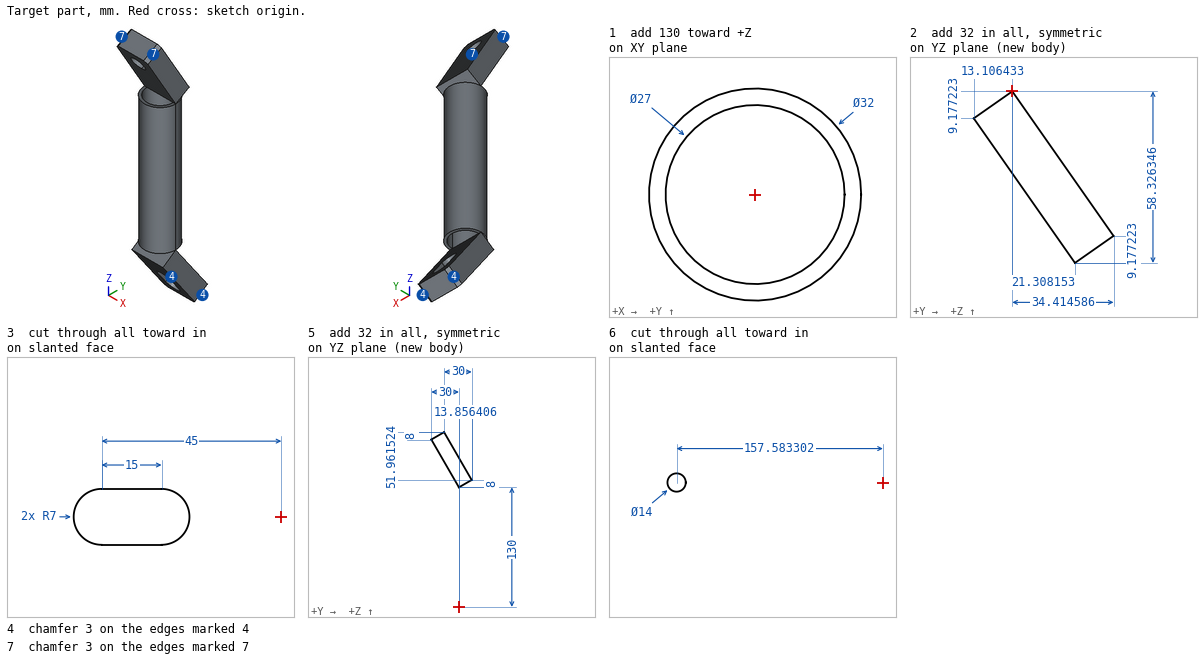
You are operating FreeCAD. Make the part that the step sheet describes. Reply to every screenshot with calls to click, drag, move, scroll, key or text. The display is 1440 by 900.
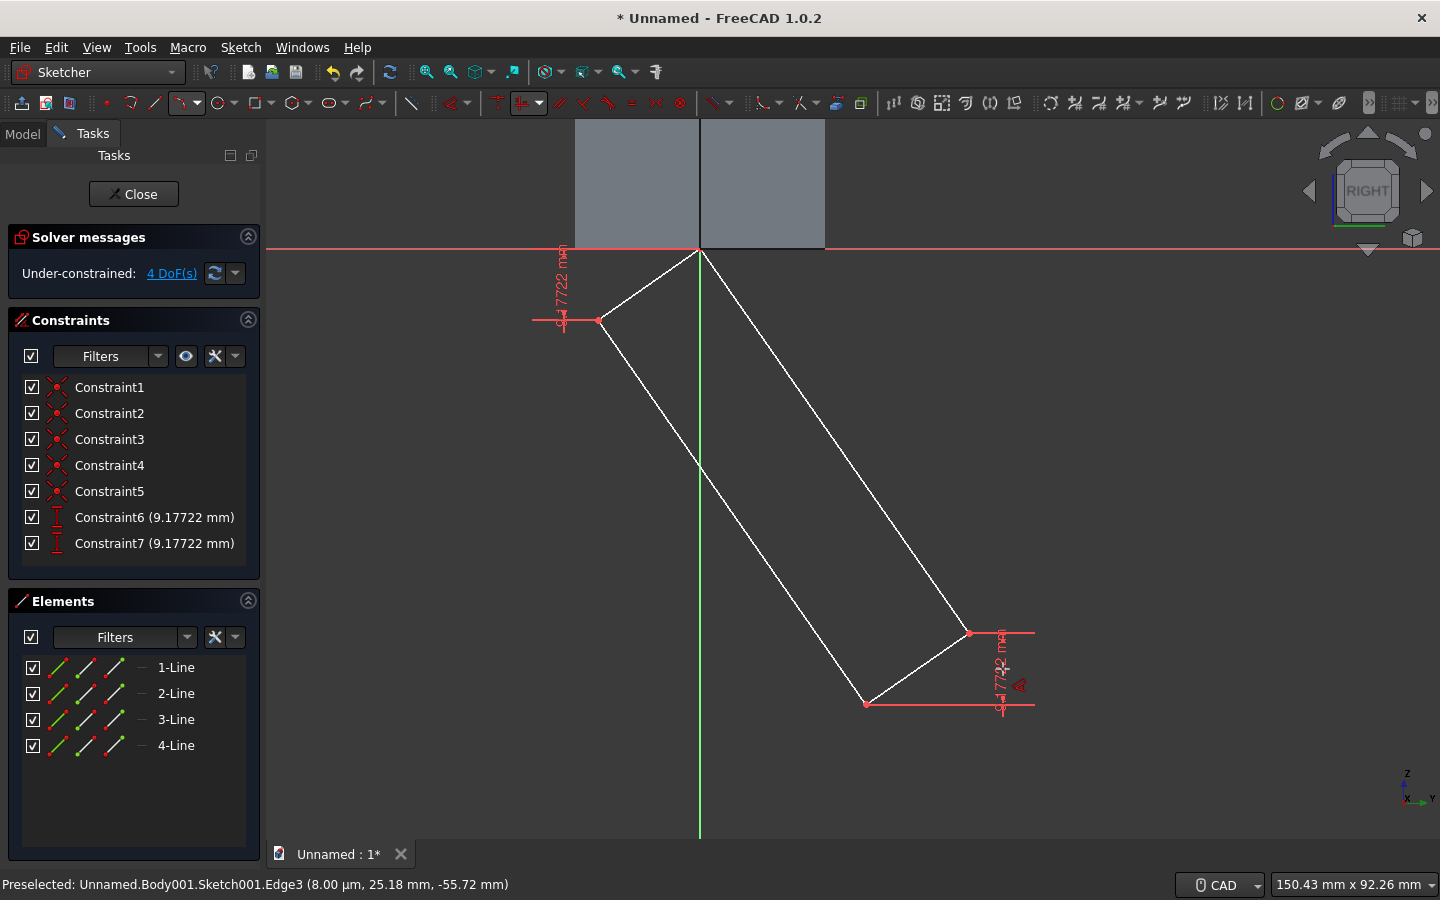
click(598, 320)
click(649, 215)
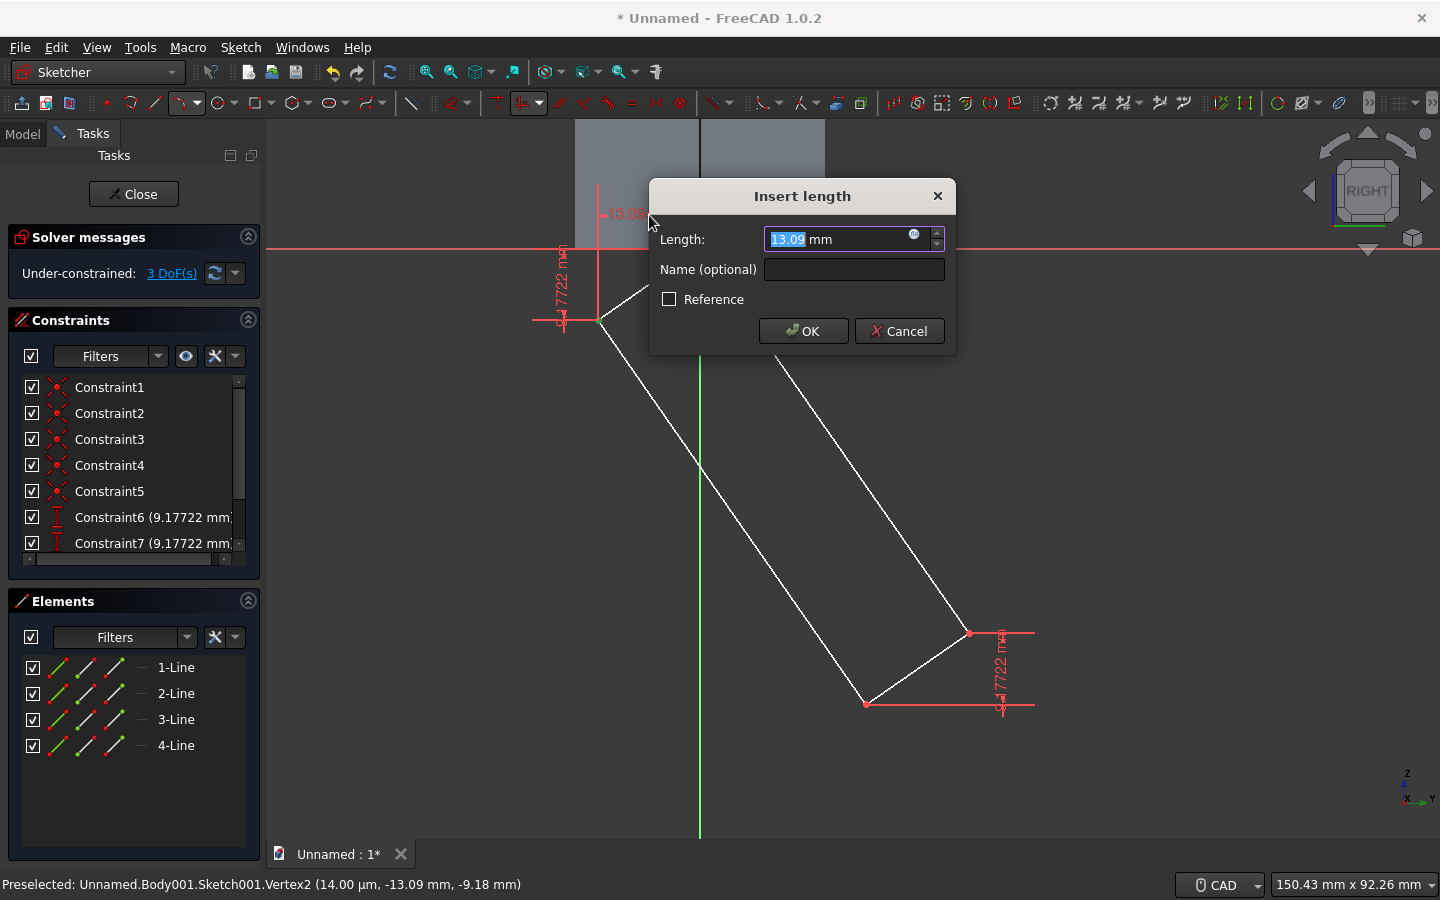
text(13.106433)
key(Return)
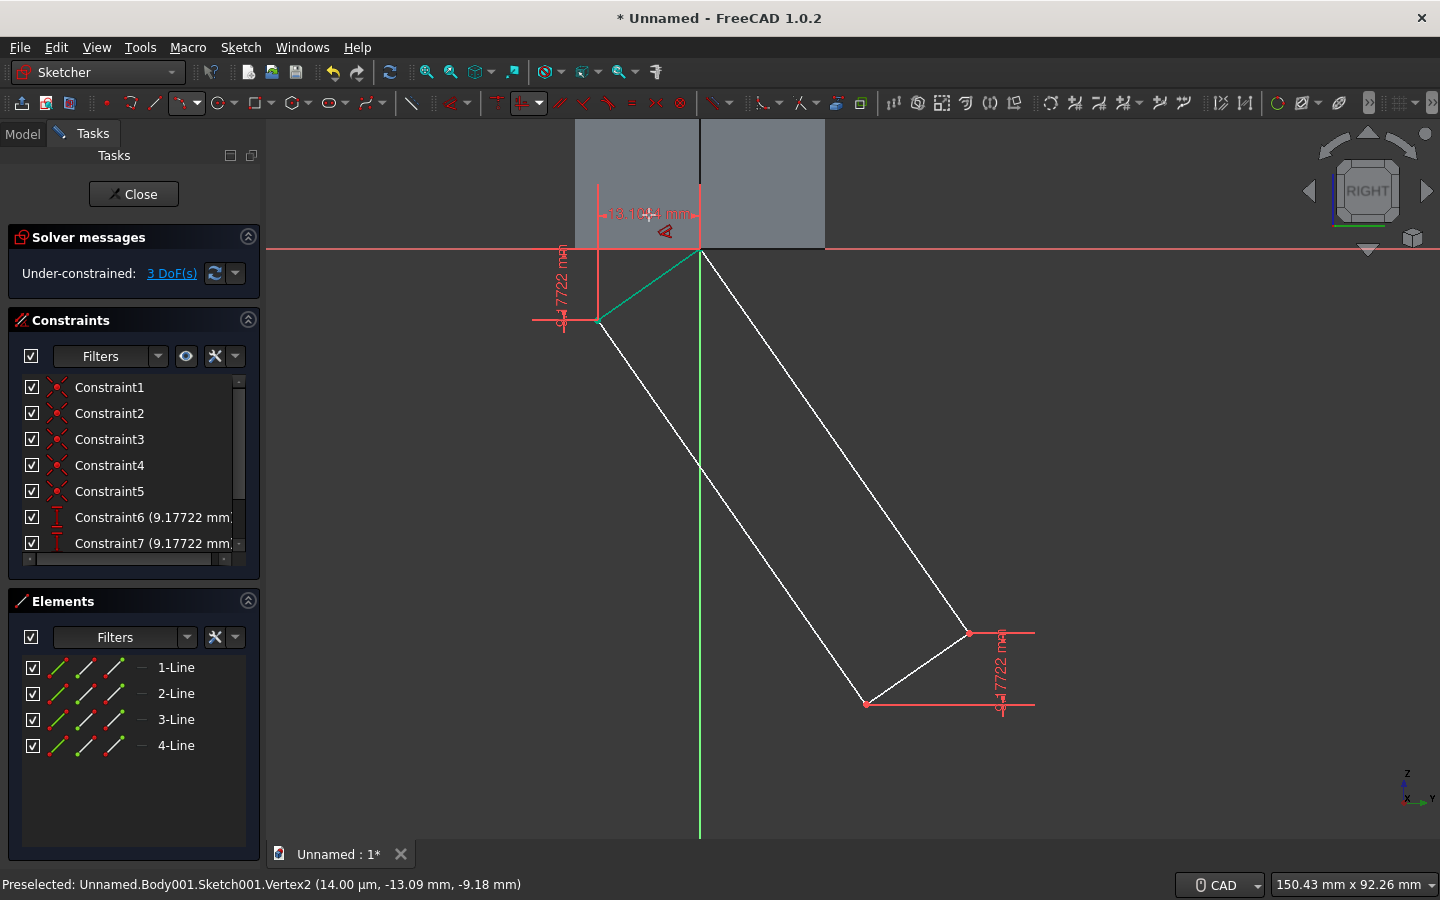
click(866, 705)
click(783, 739)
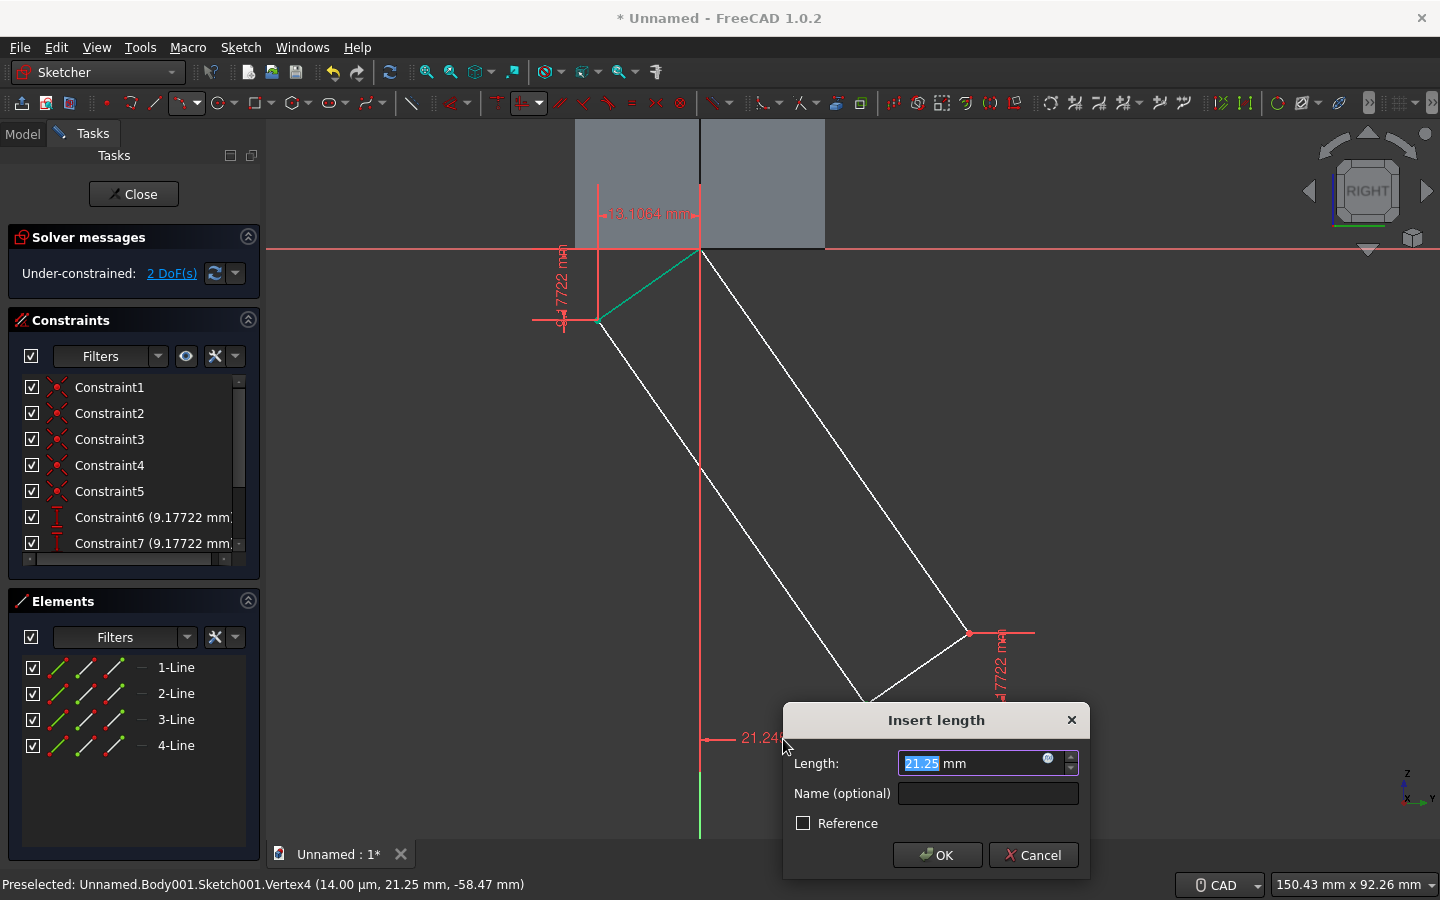
text(21.308153)
key(Return)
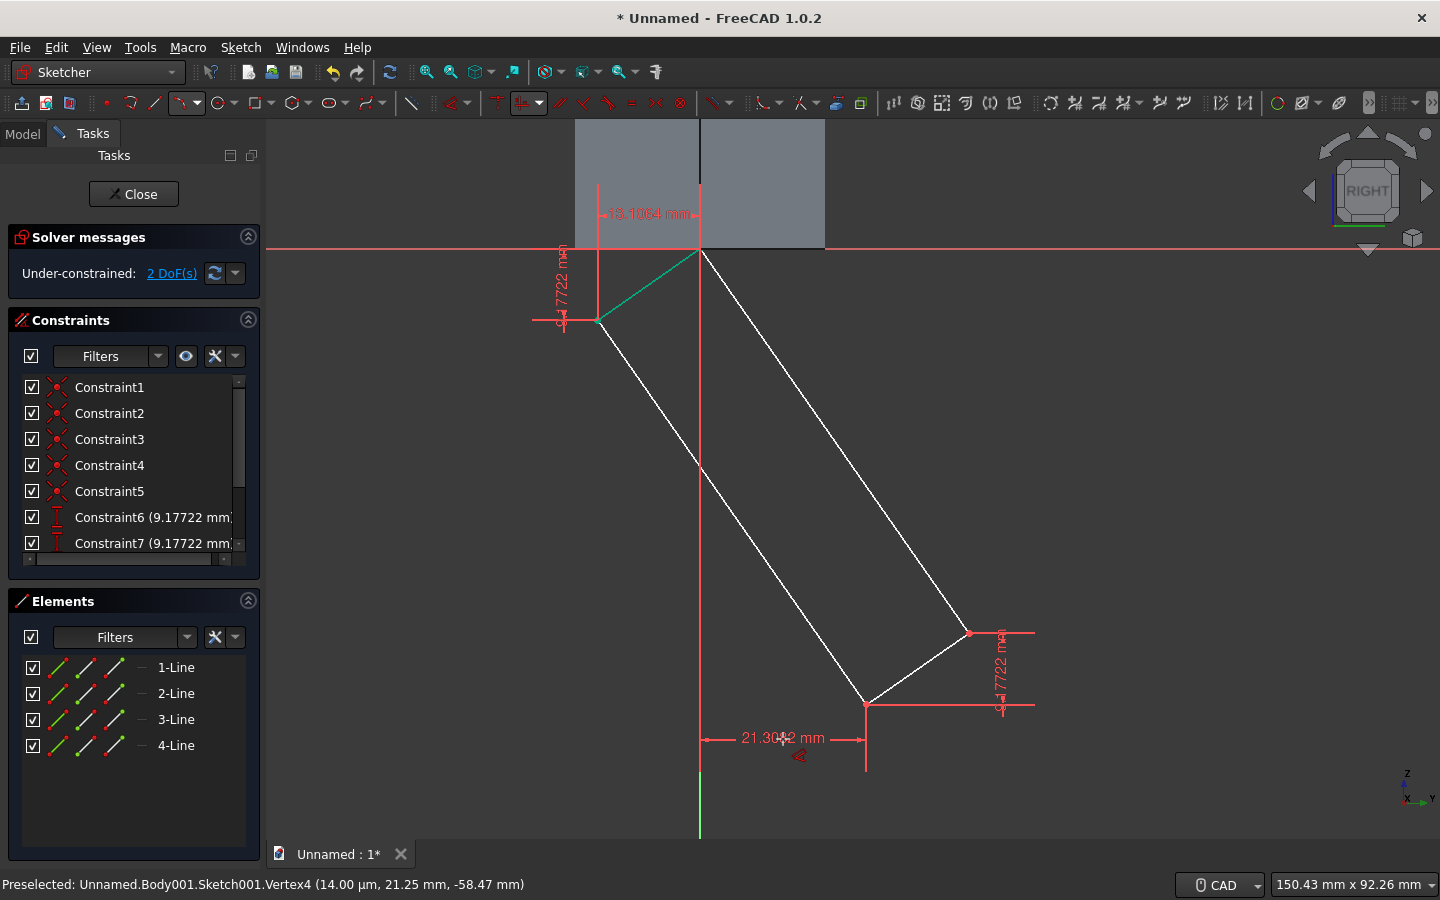
click(866, 705)
click(666, 477)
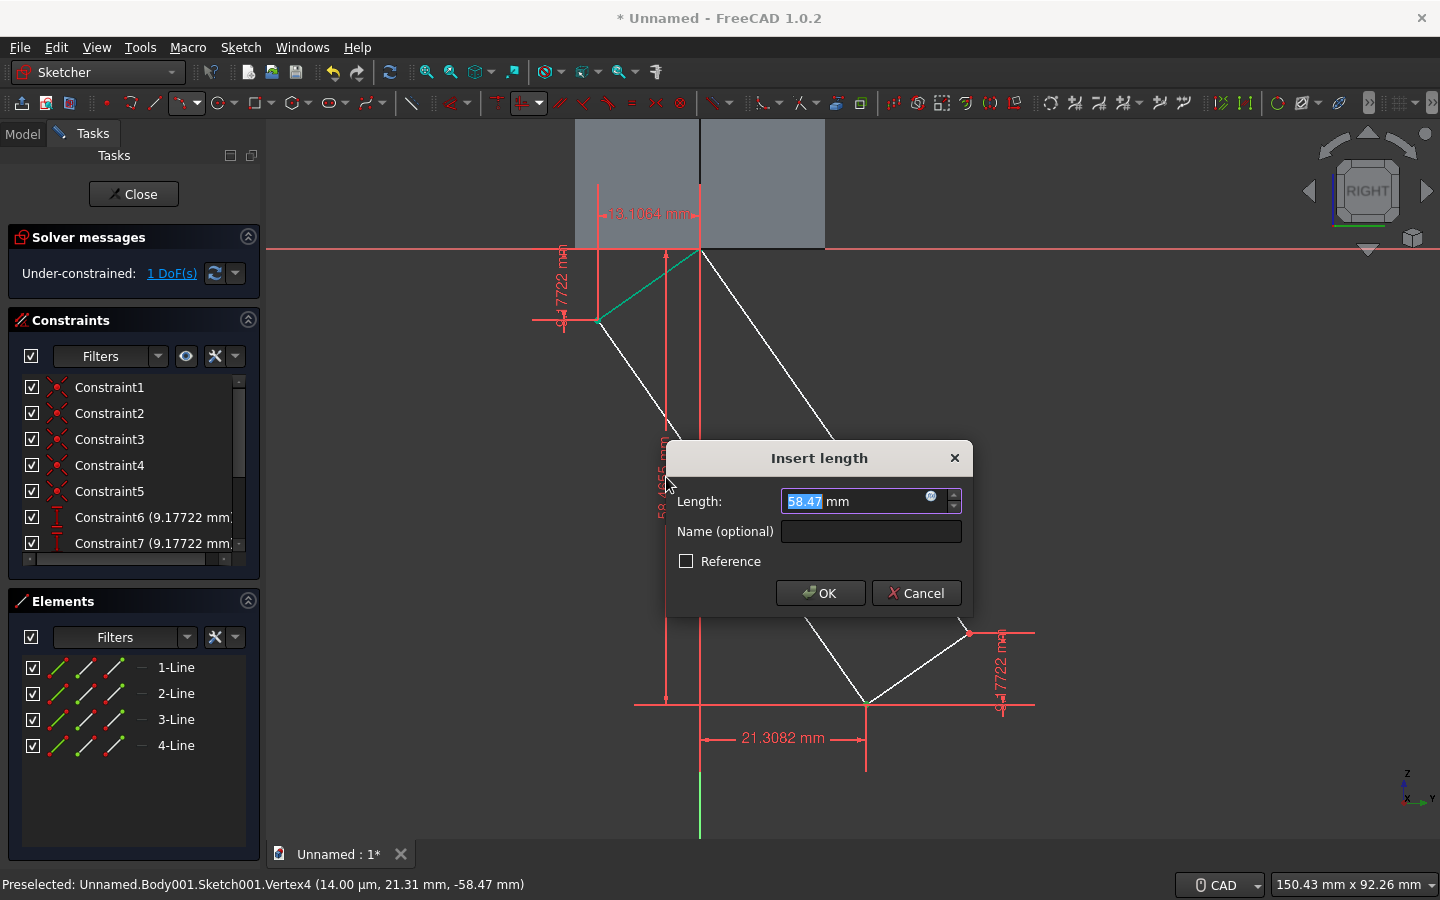
text(58.326346)
key(Return)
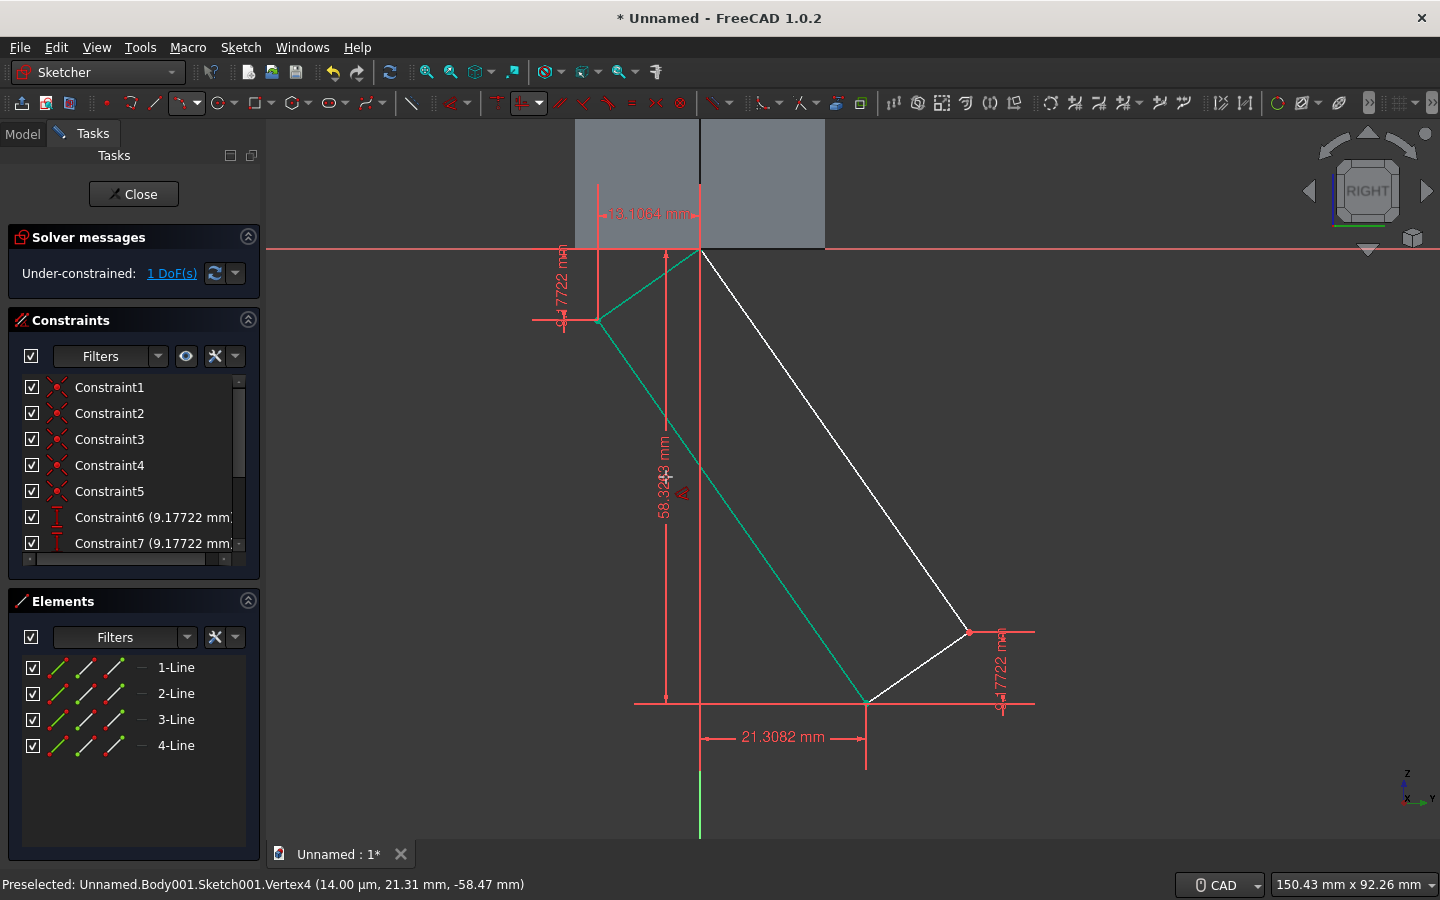
click(969, 632)
click(835, 215)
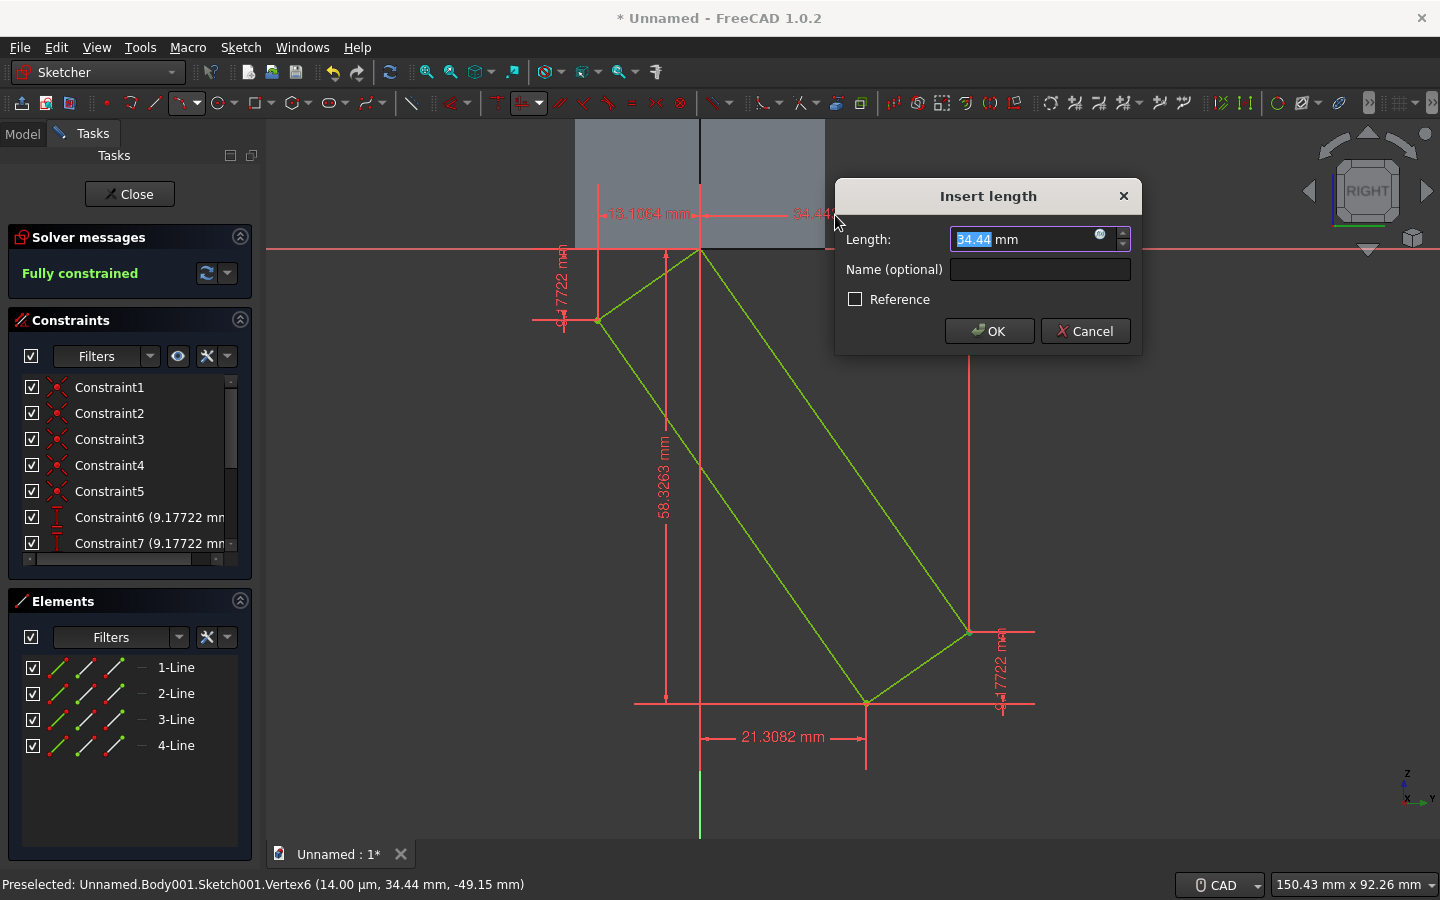
text(34.414586)
key(Return)
key(Escape)